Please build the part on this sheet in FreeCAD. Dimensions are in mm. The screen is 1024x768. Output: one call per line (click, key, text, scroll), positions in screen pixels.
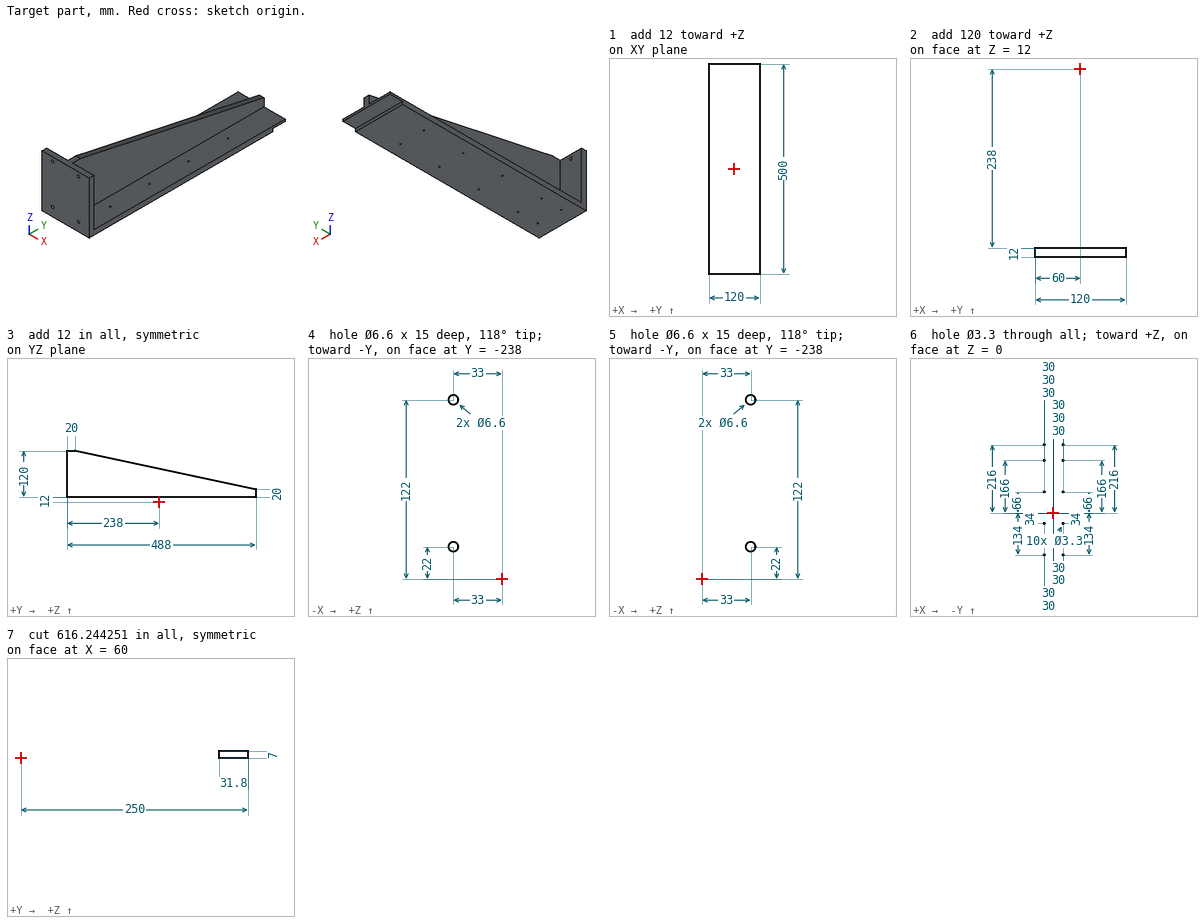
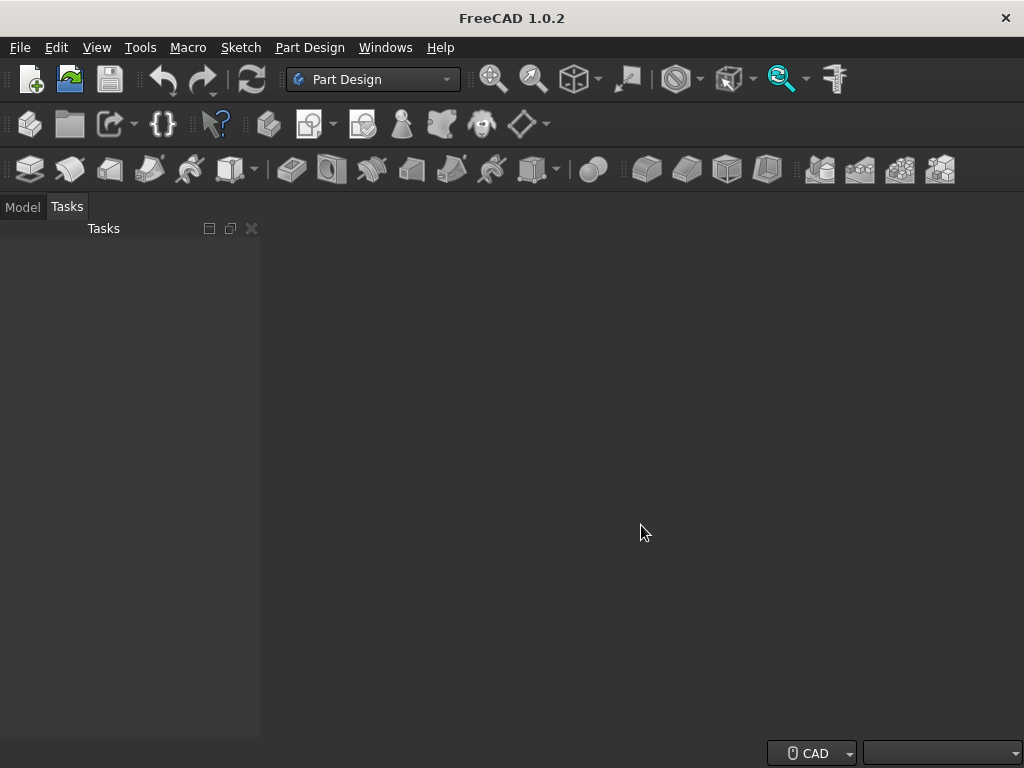
click(30, 80)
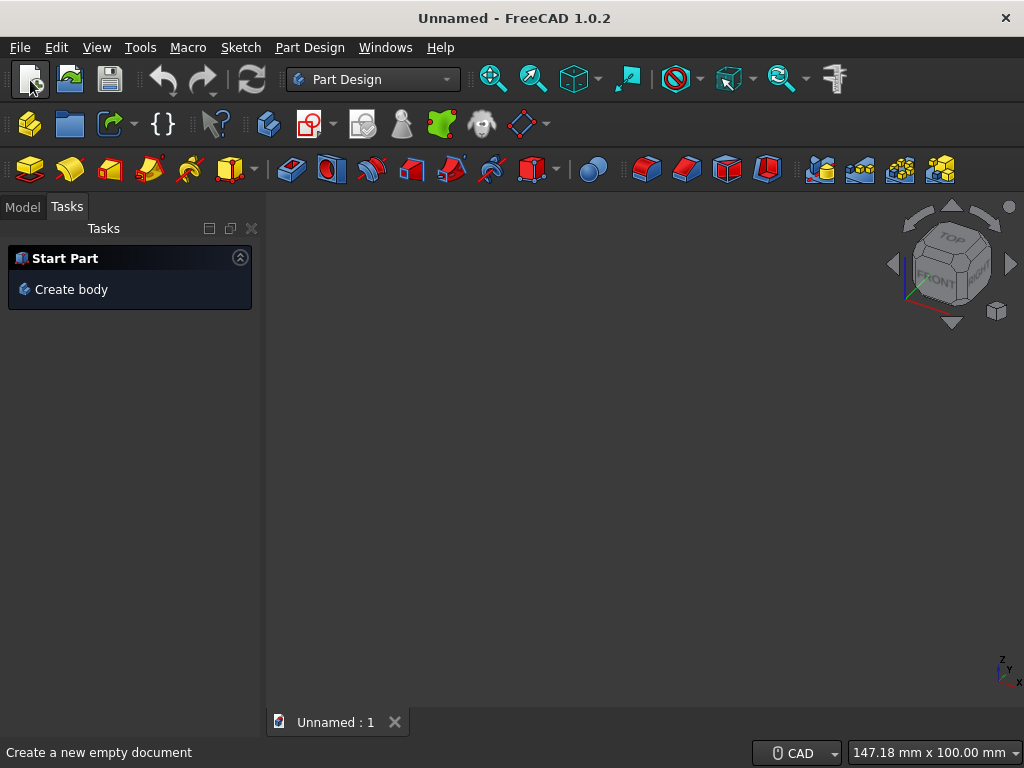
click(310, 124)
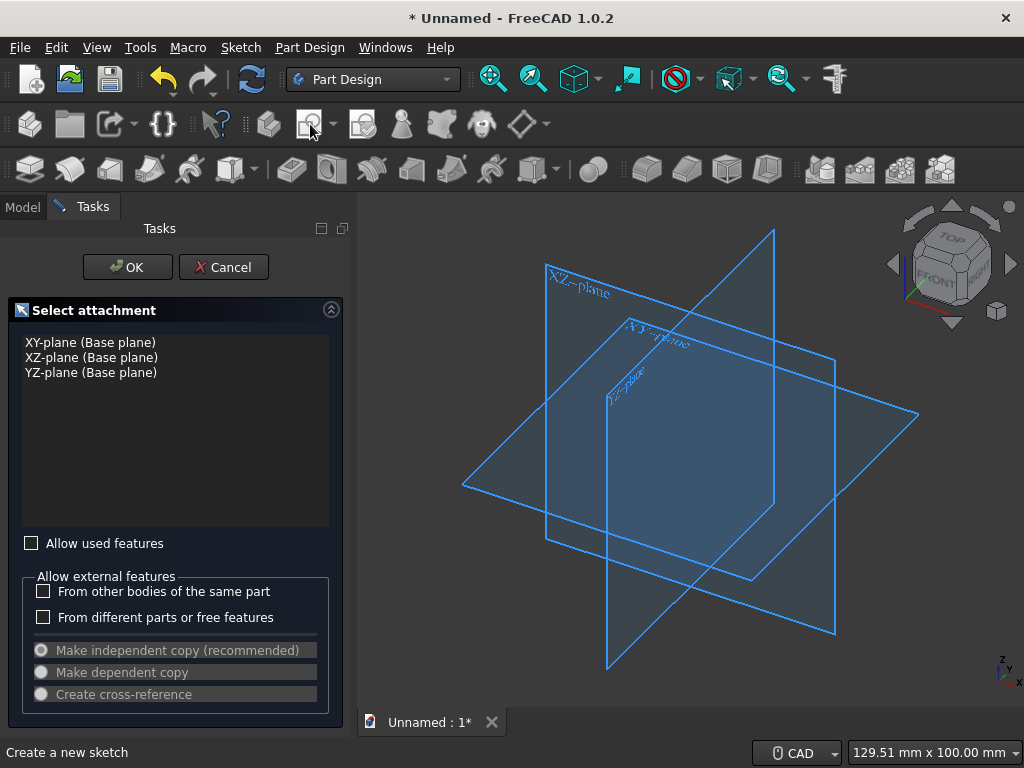
click(82, 342)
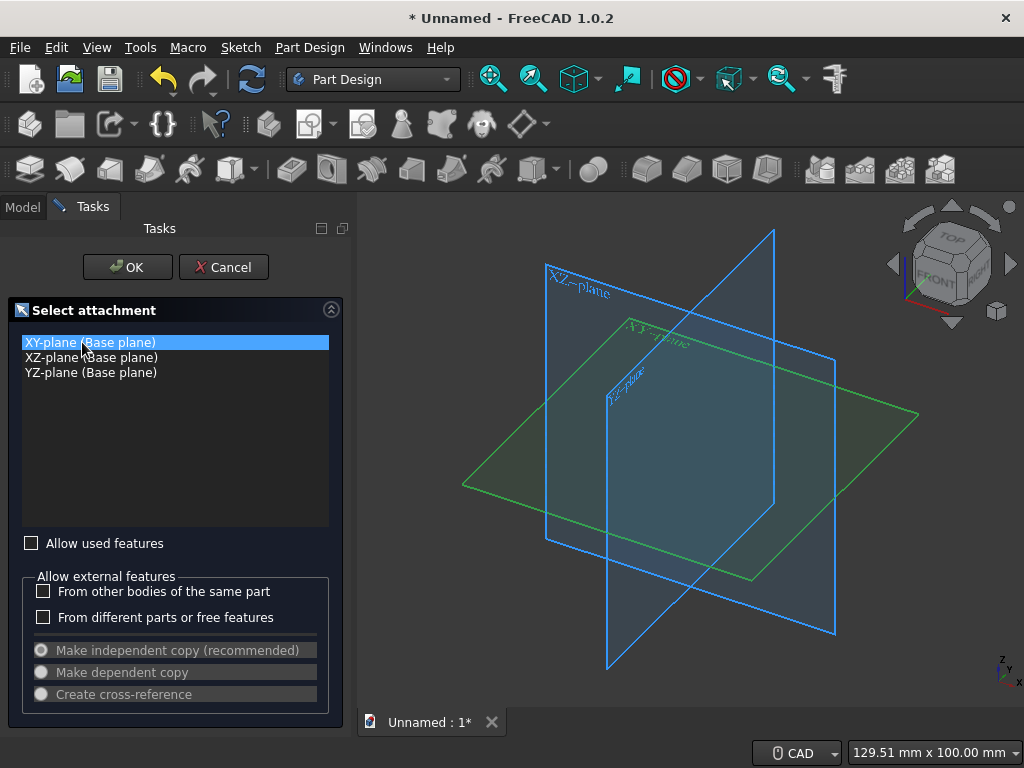
click(128, 267)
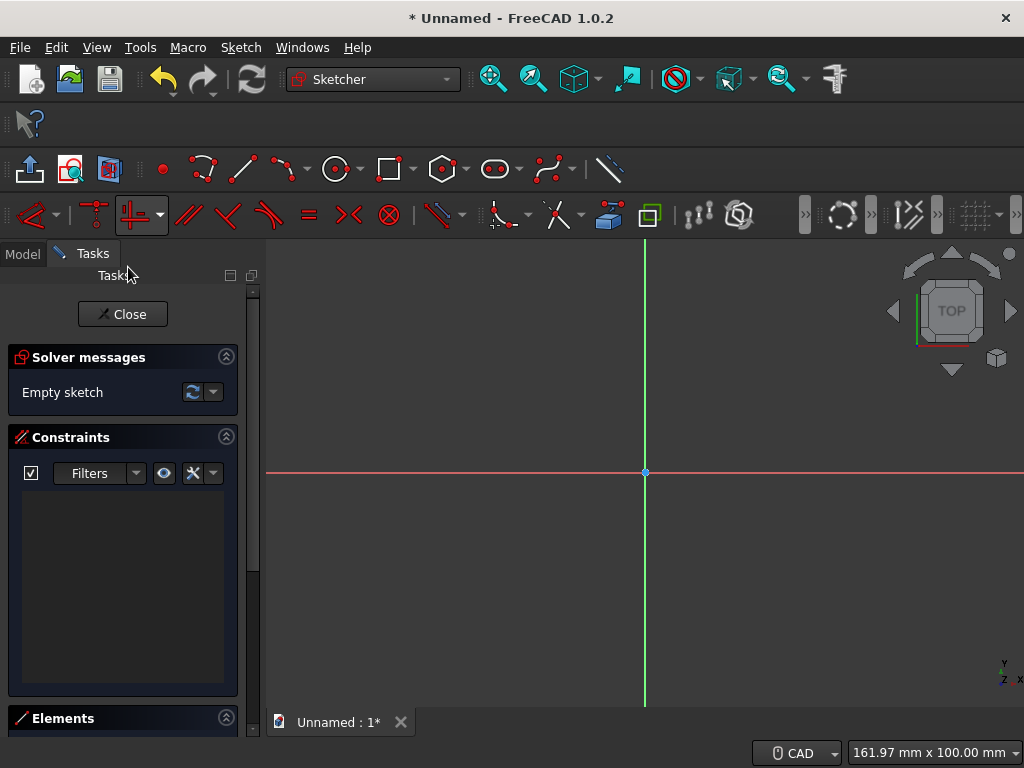
scroll(566, 473, down, 10)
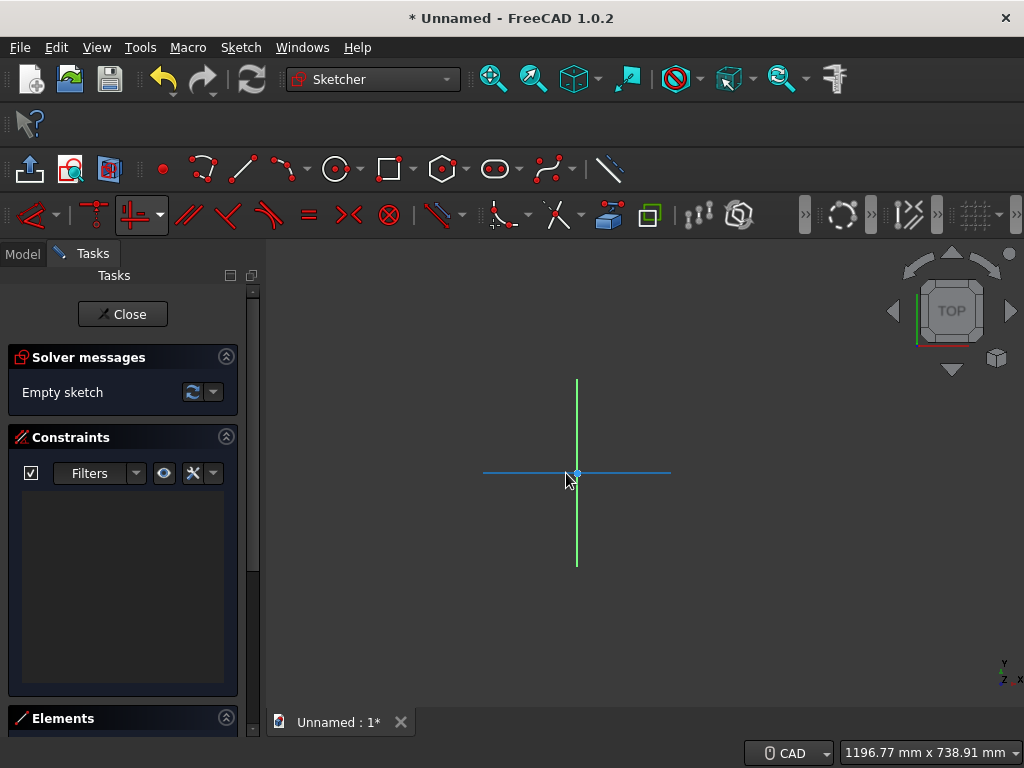
key(g)
key(v)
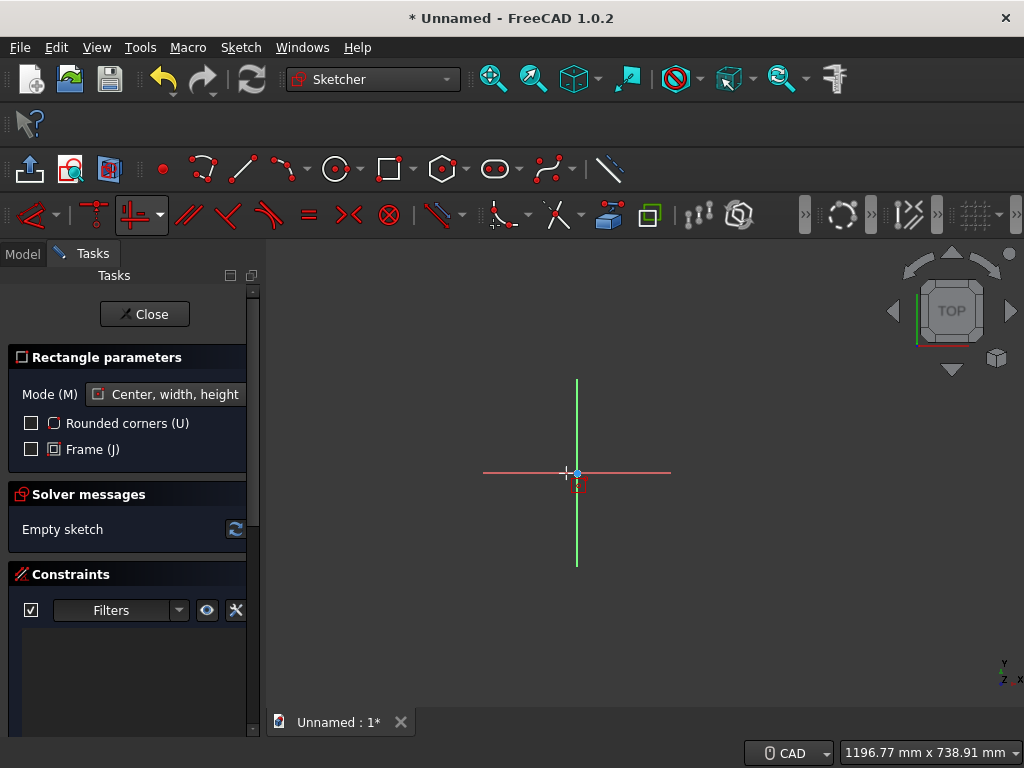
click(577, 473)
click(615, 315)
key(Escape)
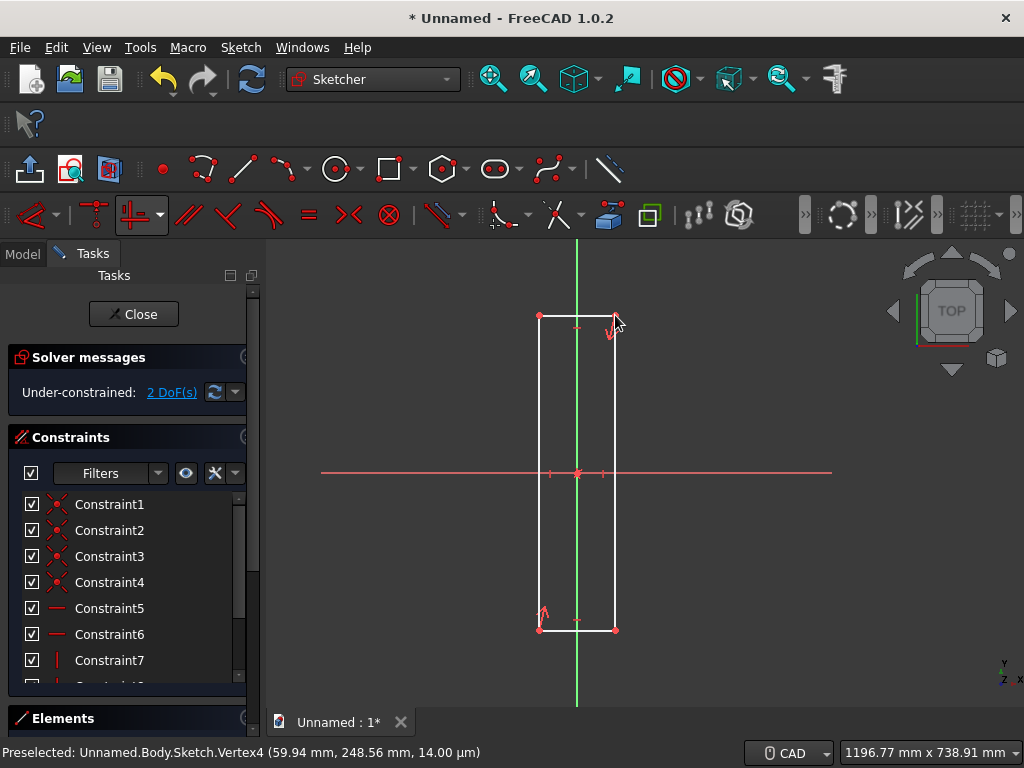
click(562, 631)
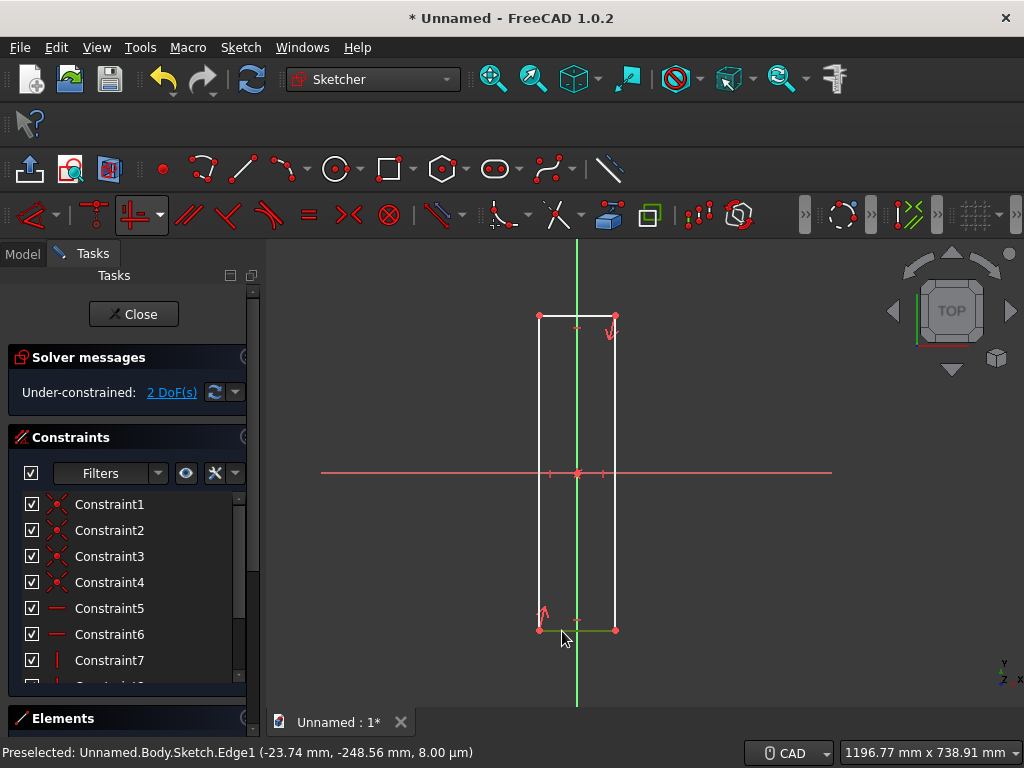
key(l)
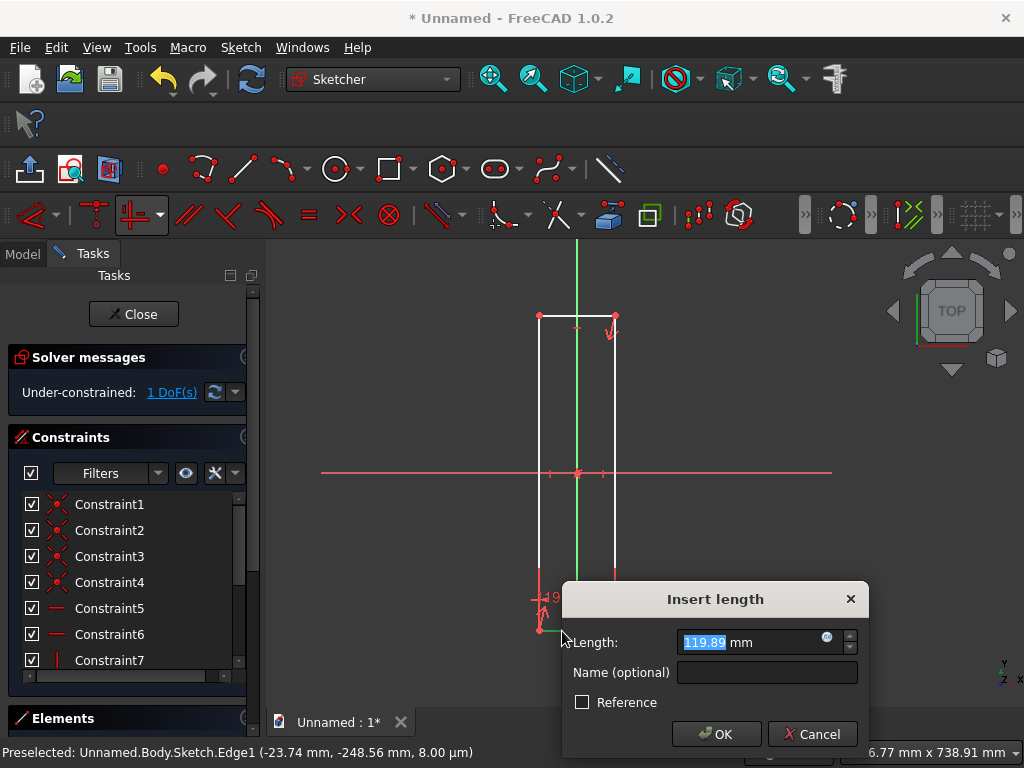
text(120)
key(Return)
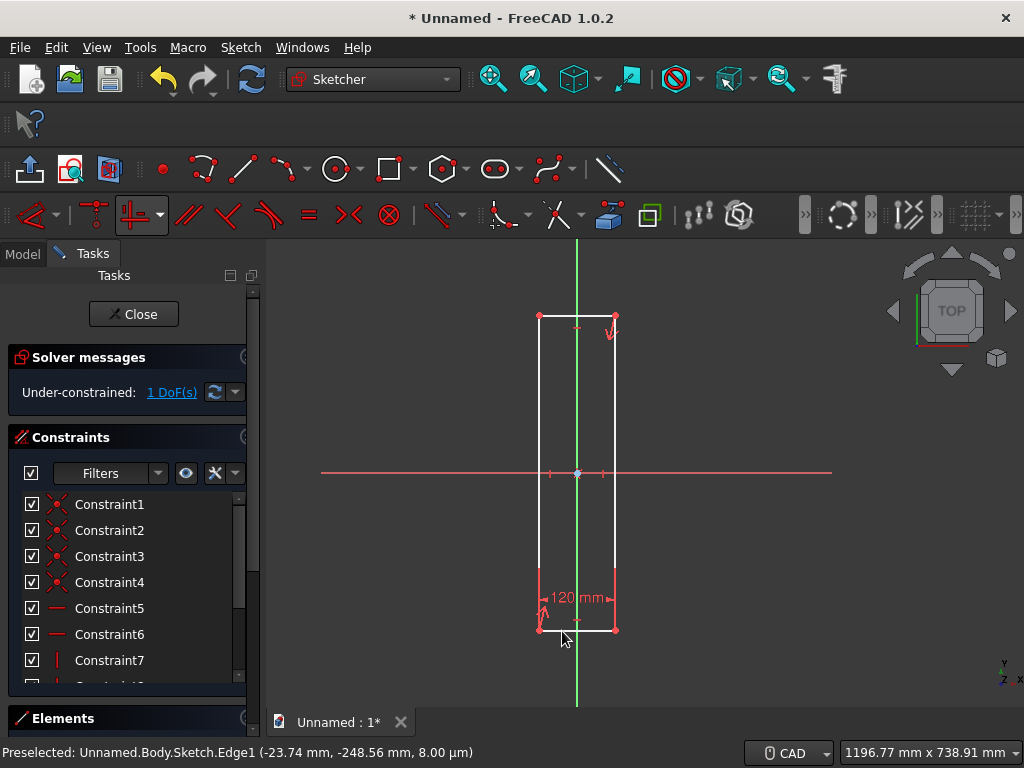
click(615, 536)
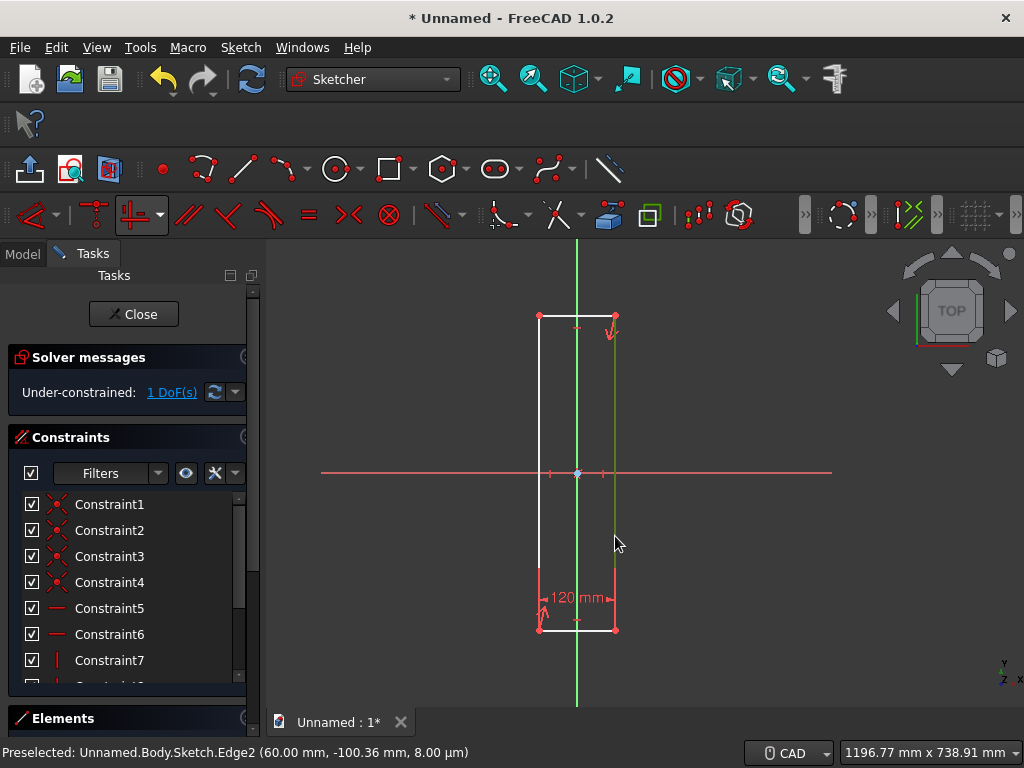
key(i)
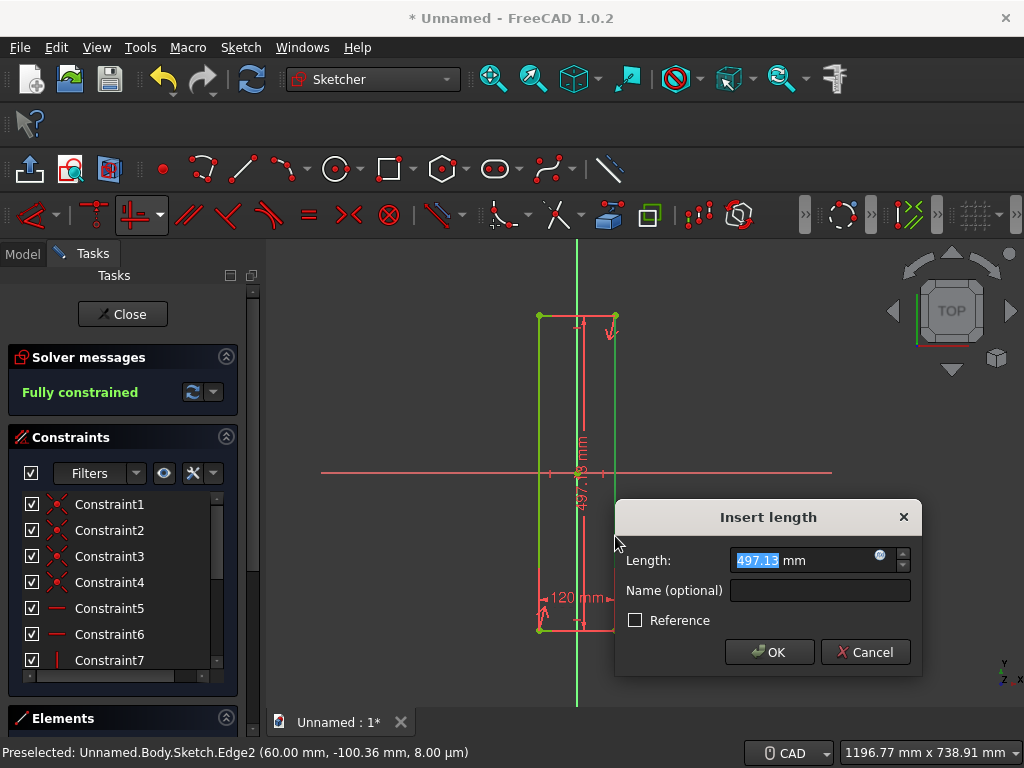
text(500)
key(Return)